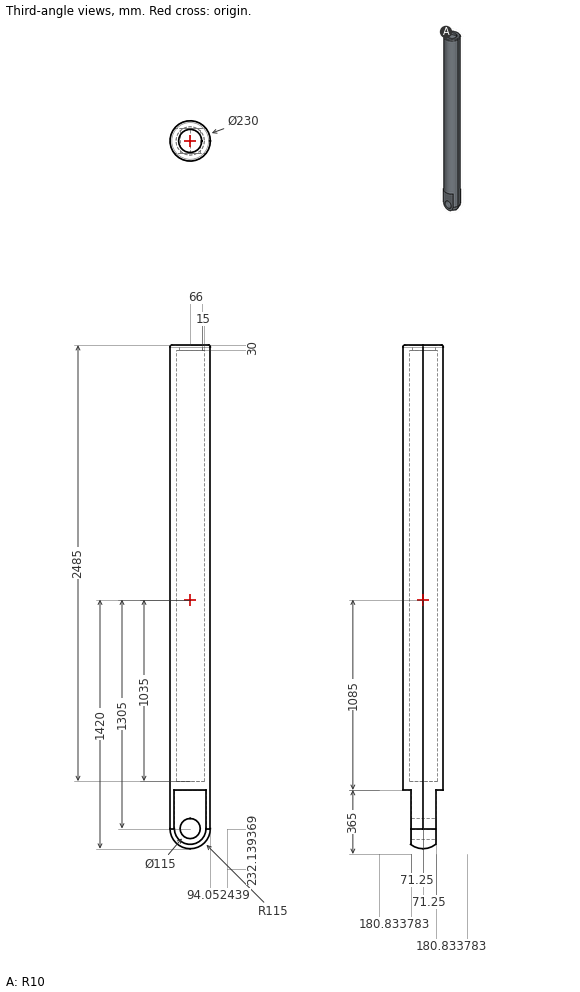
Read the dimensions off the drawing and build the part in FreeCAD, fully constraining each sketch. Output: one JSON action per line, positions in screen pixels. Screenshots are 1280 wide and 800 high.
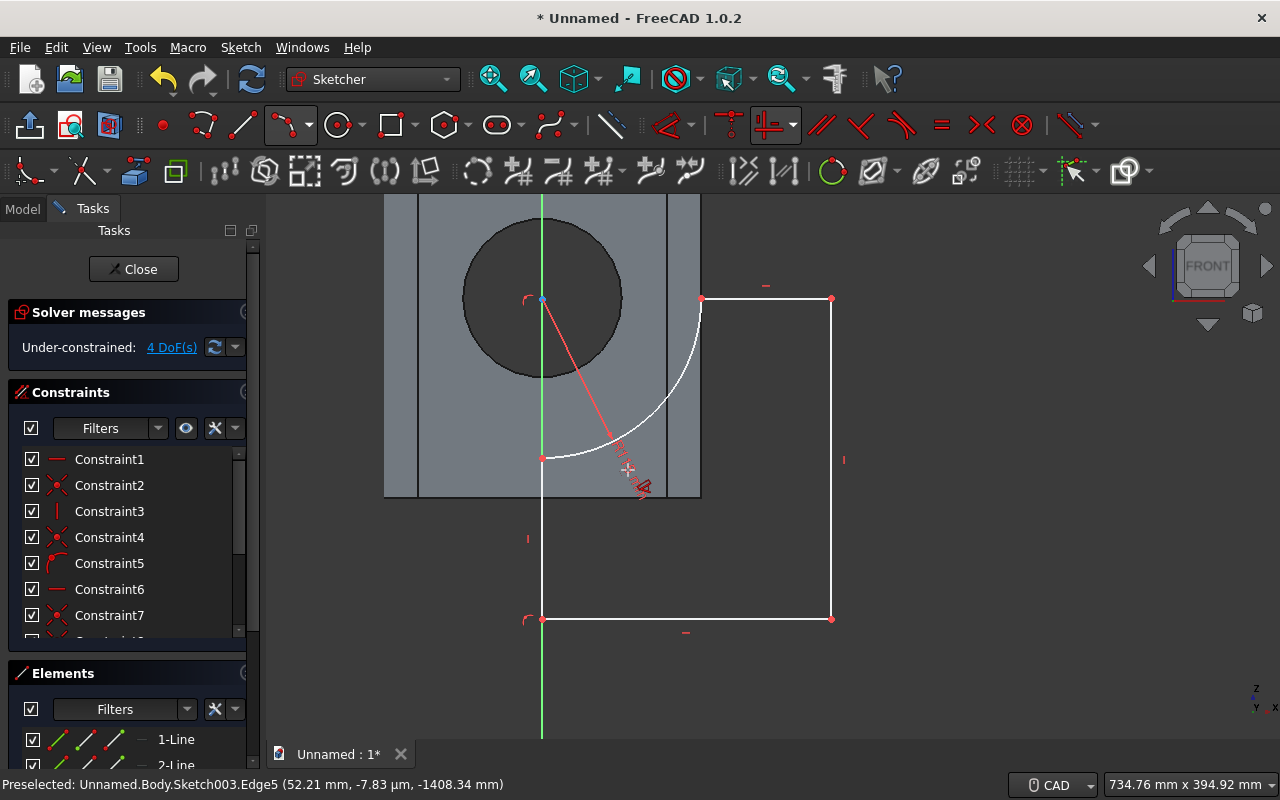
{"action": "left_click", "coordinate": [701, 299]}
{"action": "left_click", "coordinate": [508, 260]}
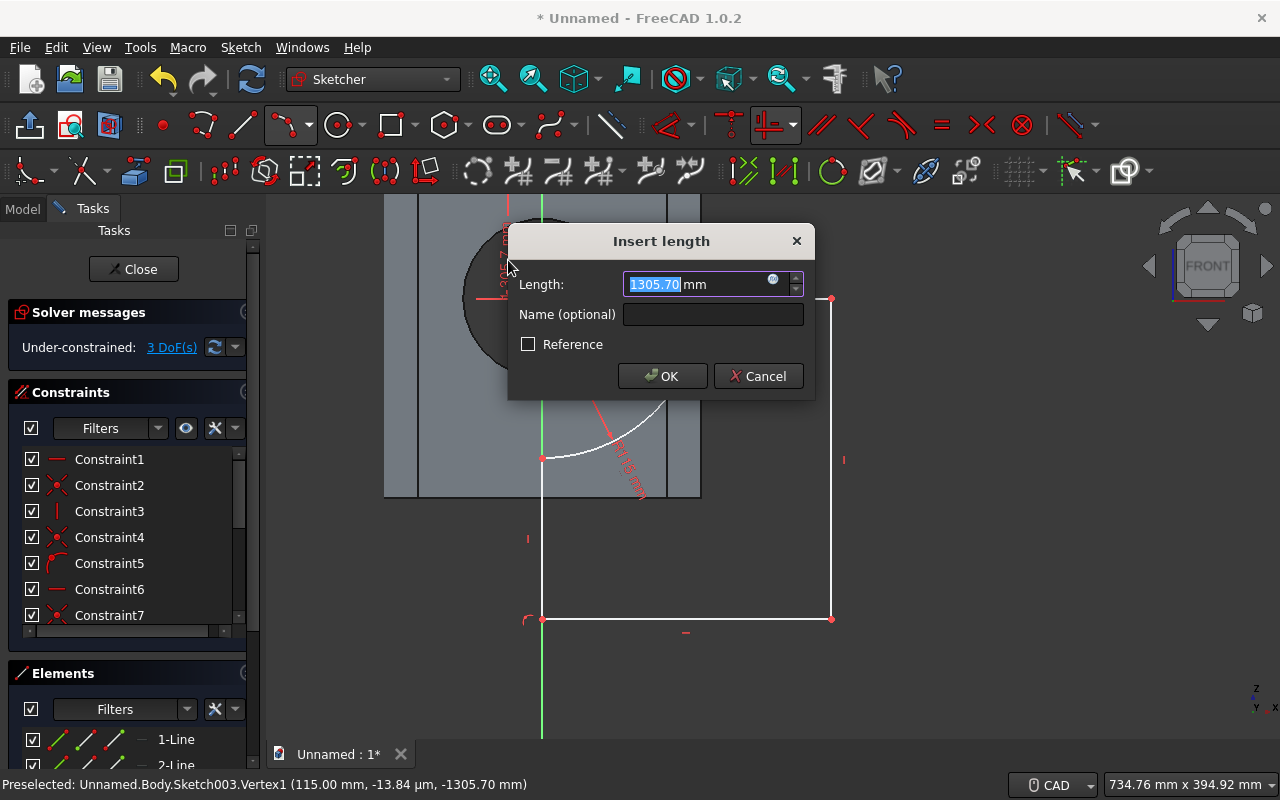
{"action": "type", "text": "1305"}
{"action": "key", "text": "Return"}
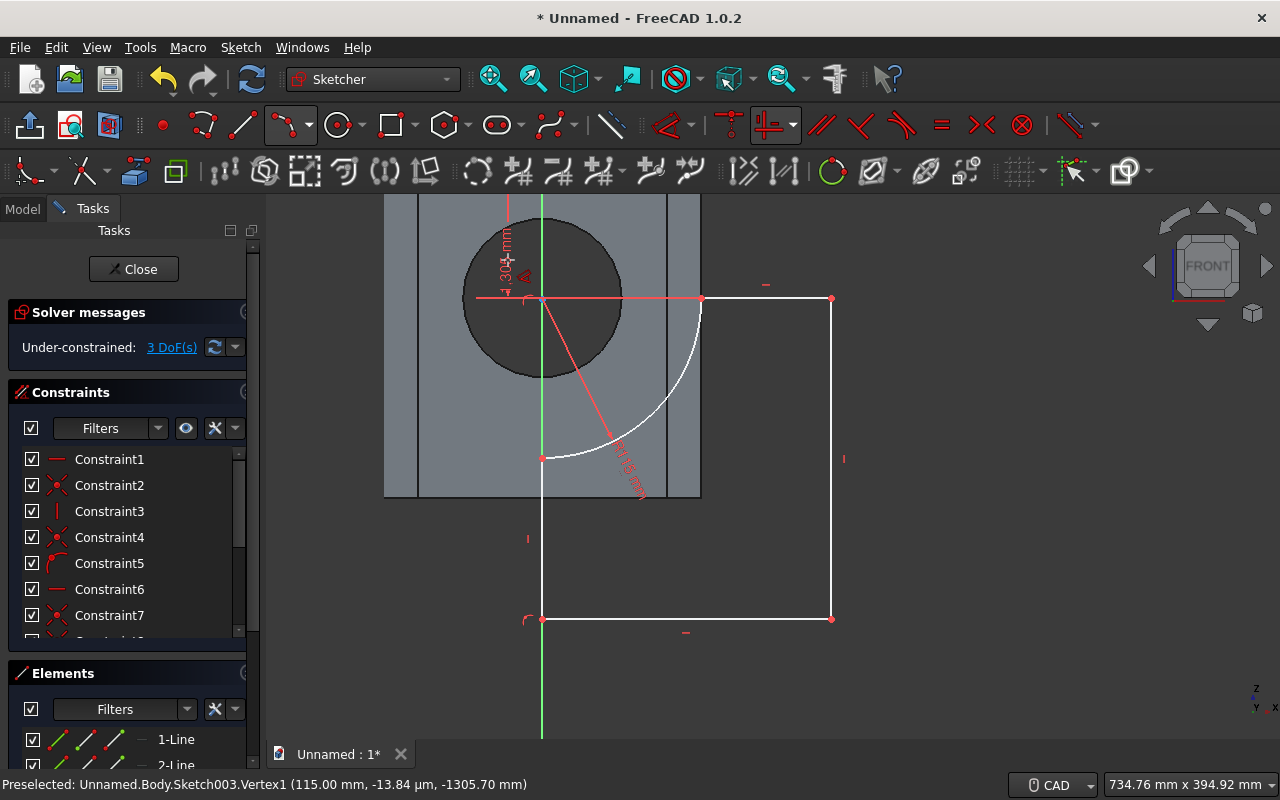
{"action": "left_click", "coordinate": [542, 458]}
{"action": "left_click", "coordinate": [508, 340]}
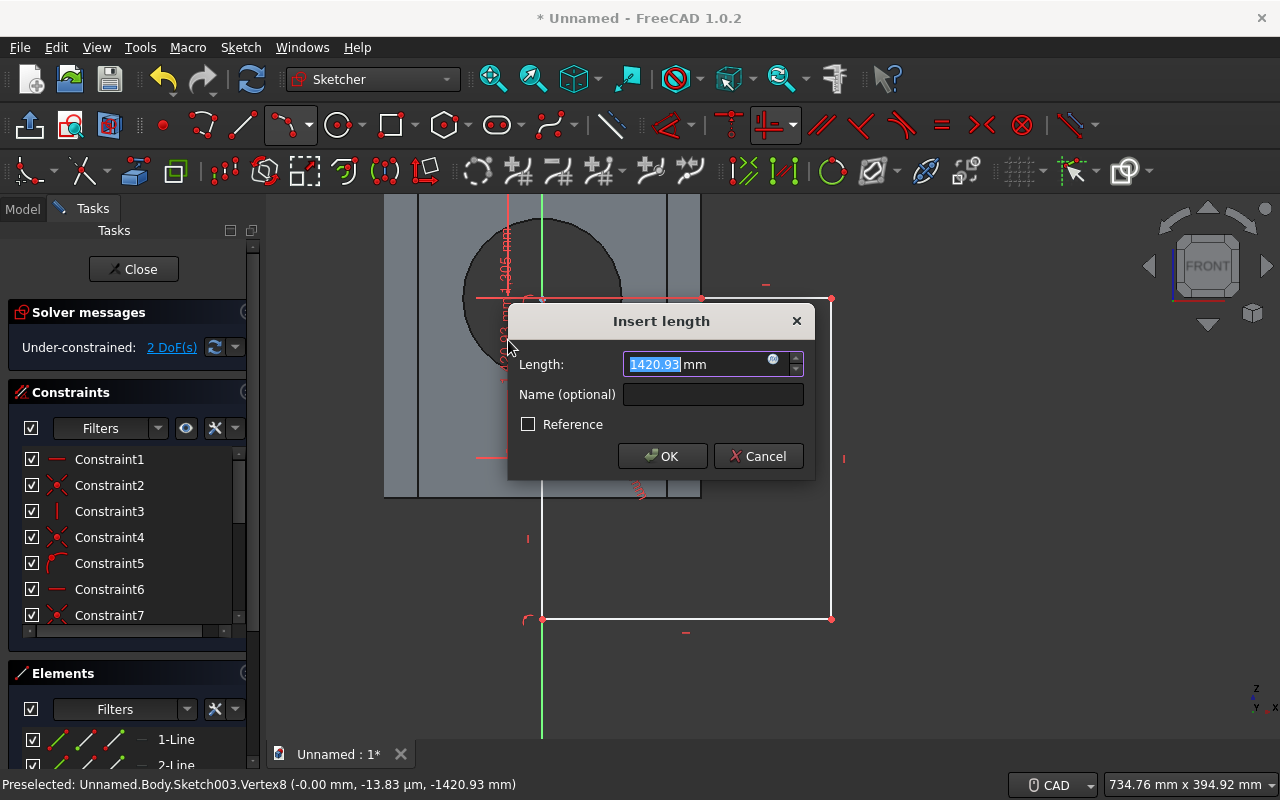
{"action": "type", "text": "1420"}
{"action": "key", "text": "Return"}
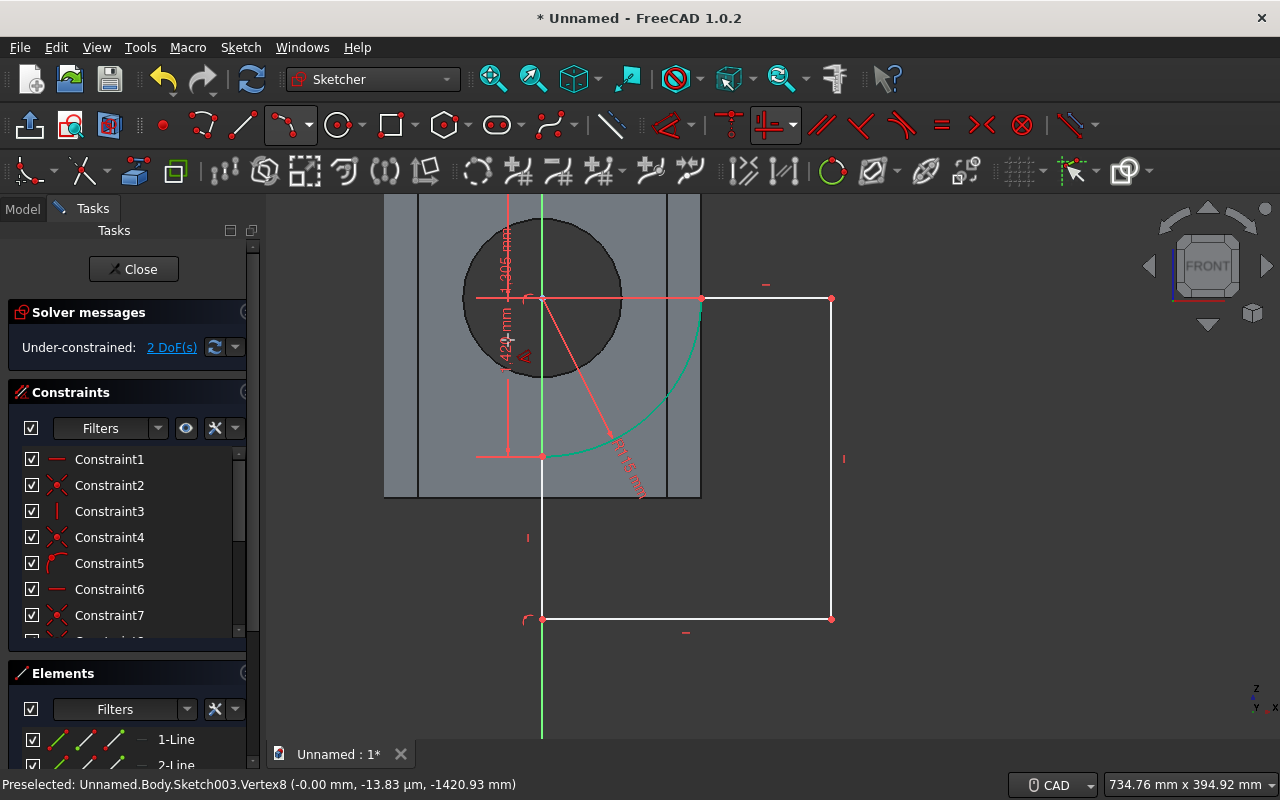
{"action": "left_click", "coordinate": [740, 298]}
{"action": "left_click", "coordinate": [766, 264]}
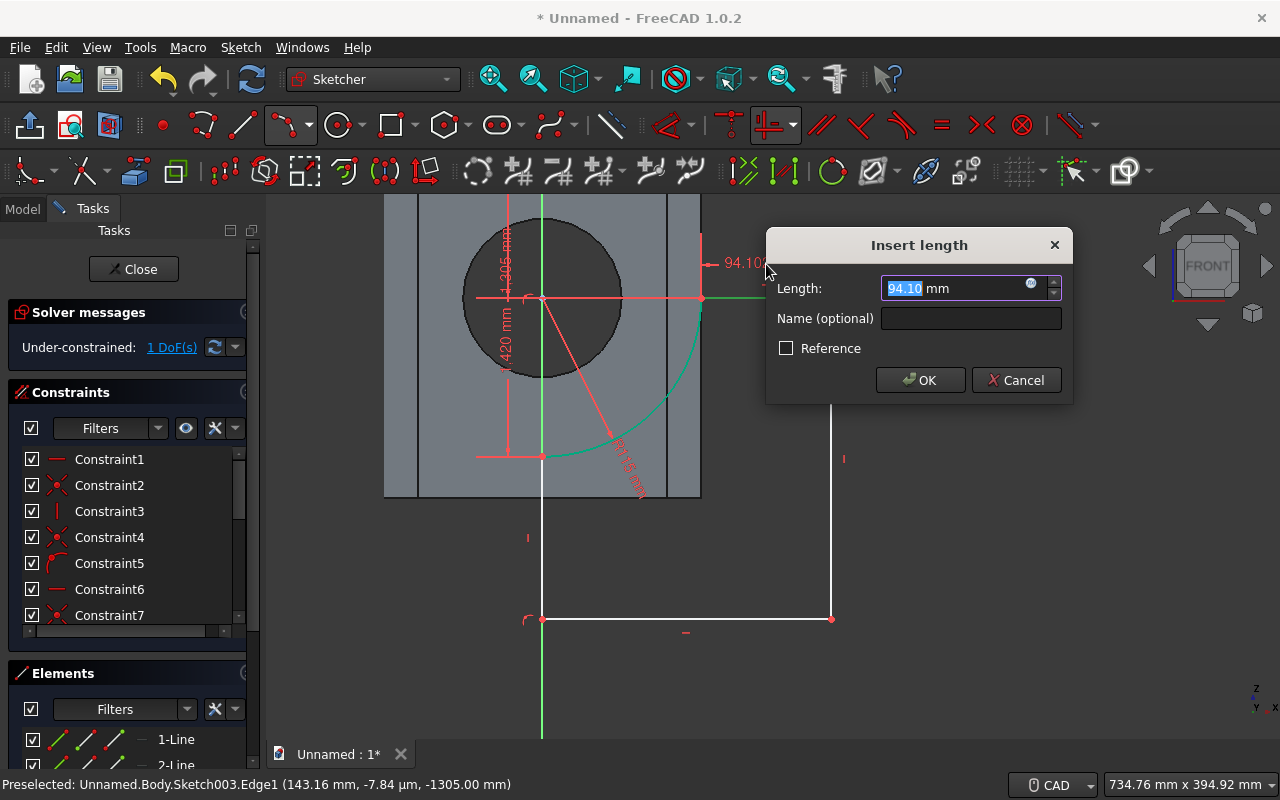
{"action": "type", "text": "94.052439"}
{"action": "key", "text": "Return"}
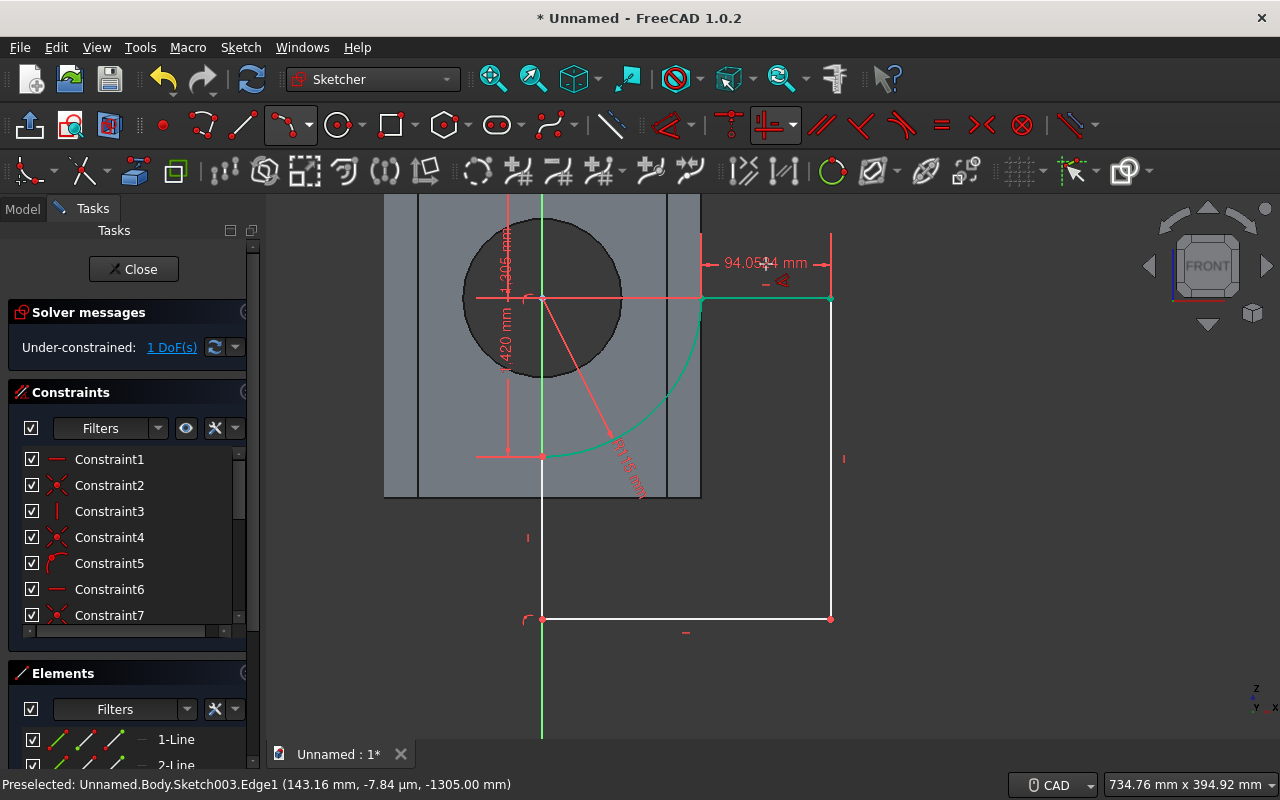
{"action": "left_click", "coordinate": [831, 394]}
{"action": "left_click", "coordinate": [865, 459]}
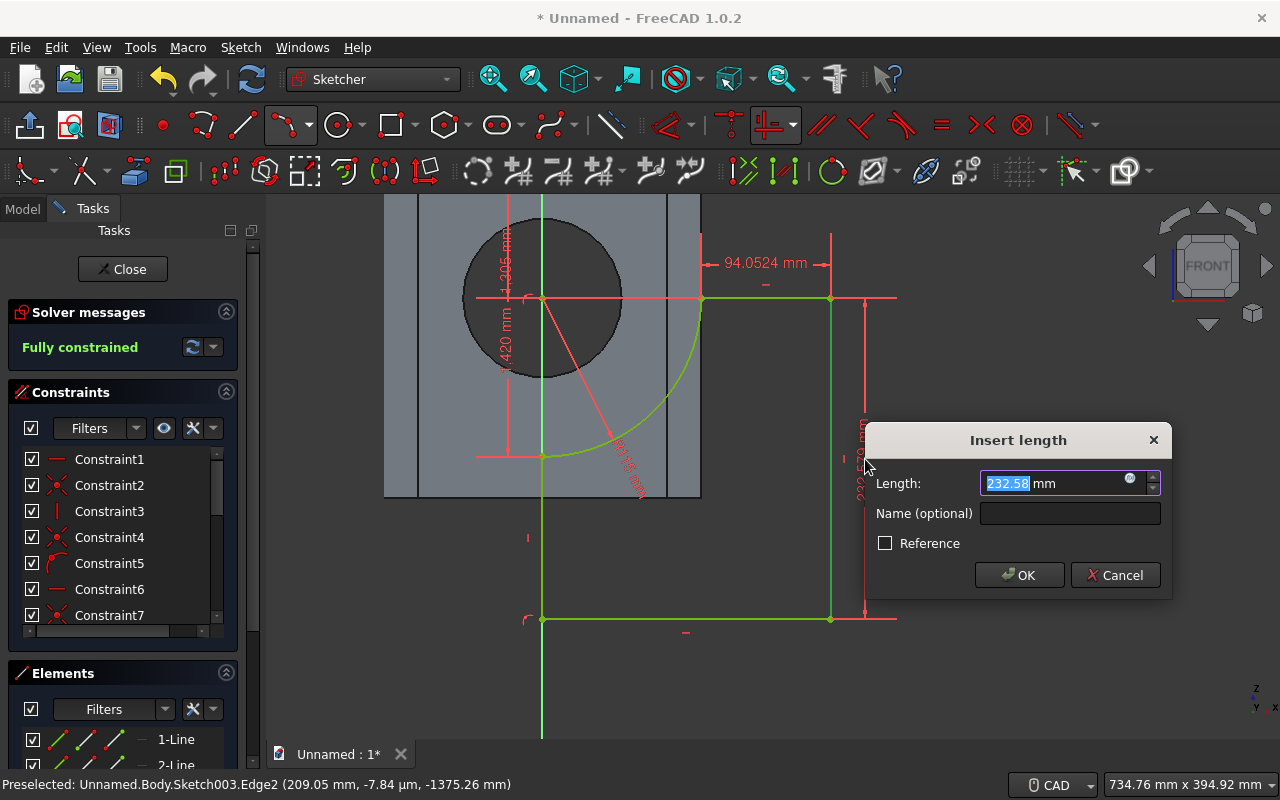
{"action": "type", "text": "232.139369"}
{"action": "key", "text": "Return"}
{"action": "key", "text": "Escape"}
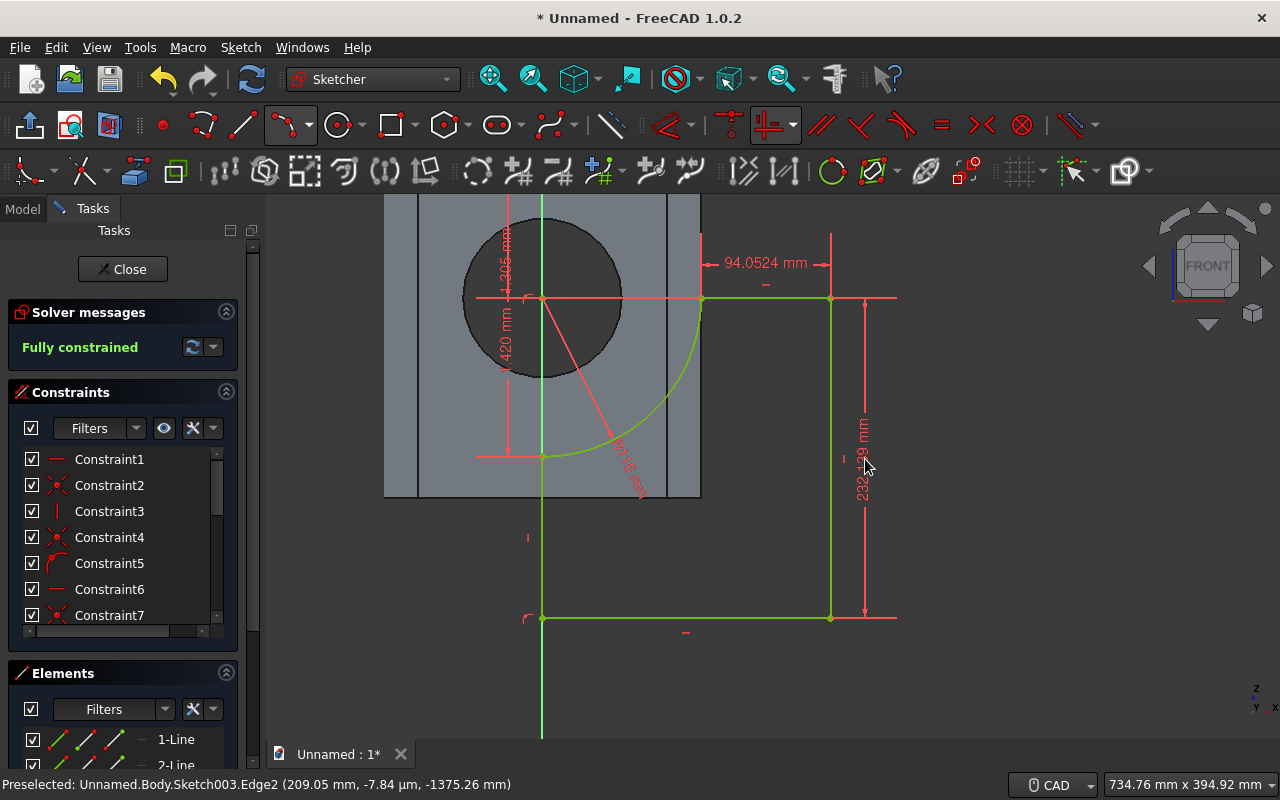
{"action": "left_click", "coordinate": [123, 269]}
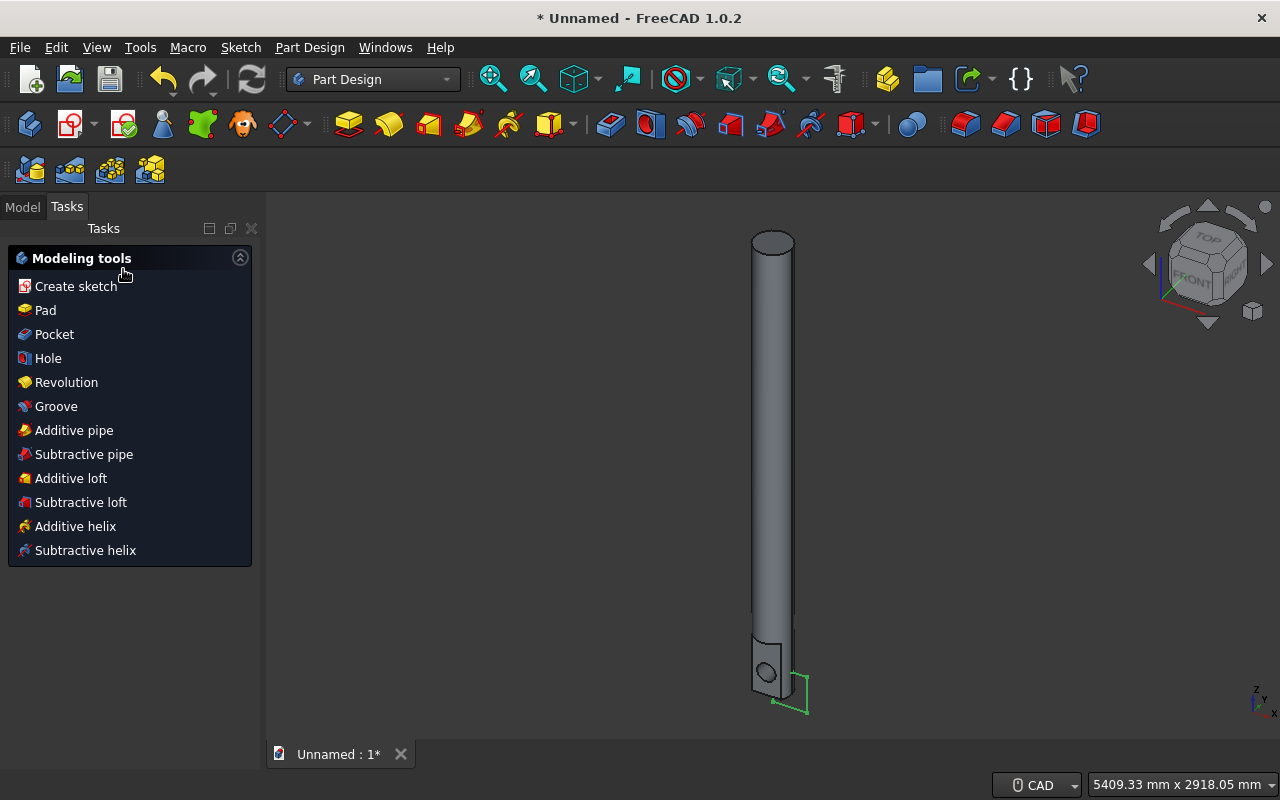
{"action": "left_click", "coordinate": [692, 124]}